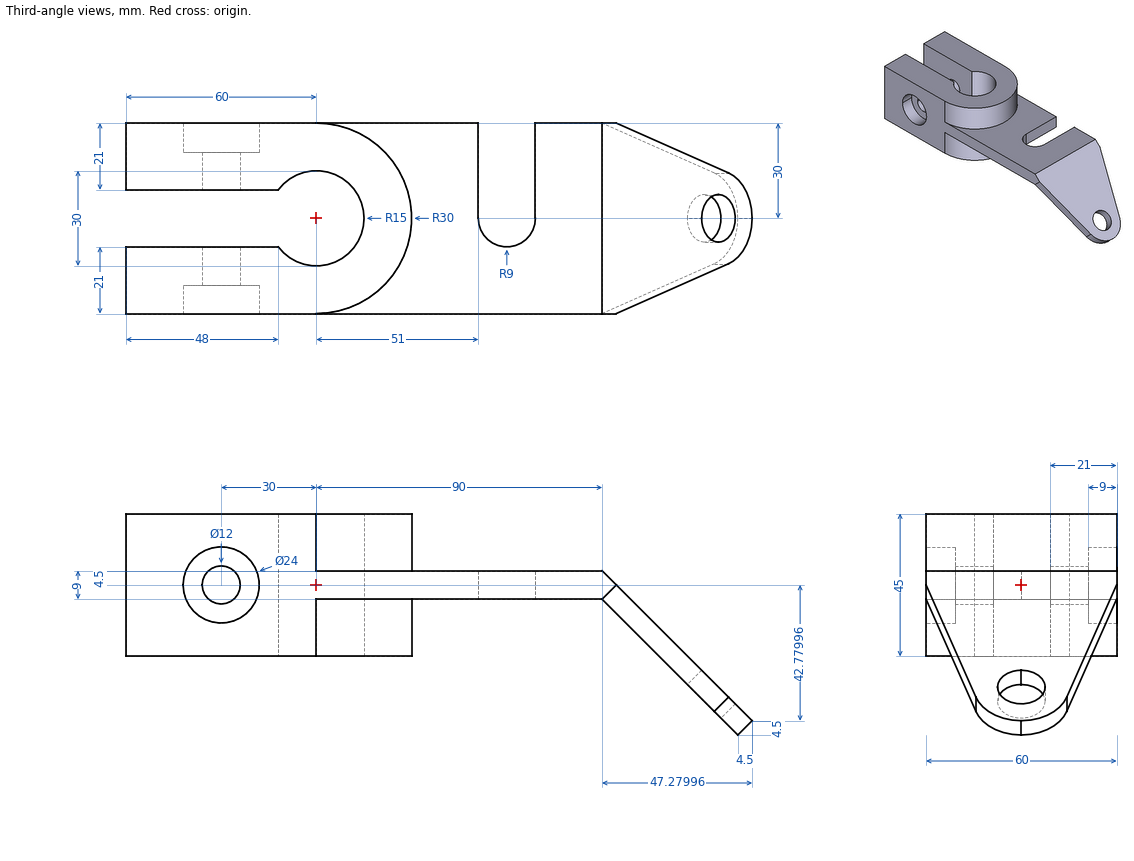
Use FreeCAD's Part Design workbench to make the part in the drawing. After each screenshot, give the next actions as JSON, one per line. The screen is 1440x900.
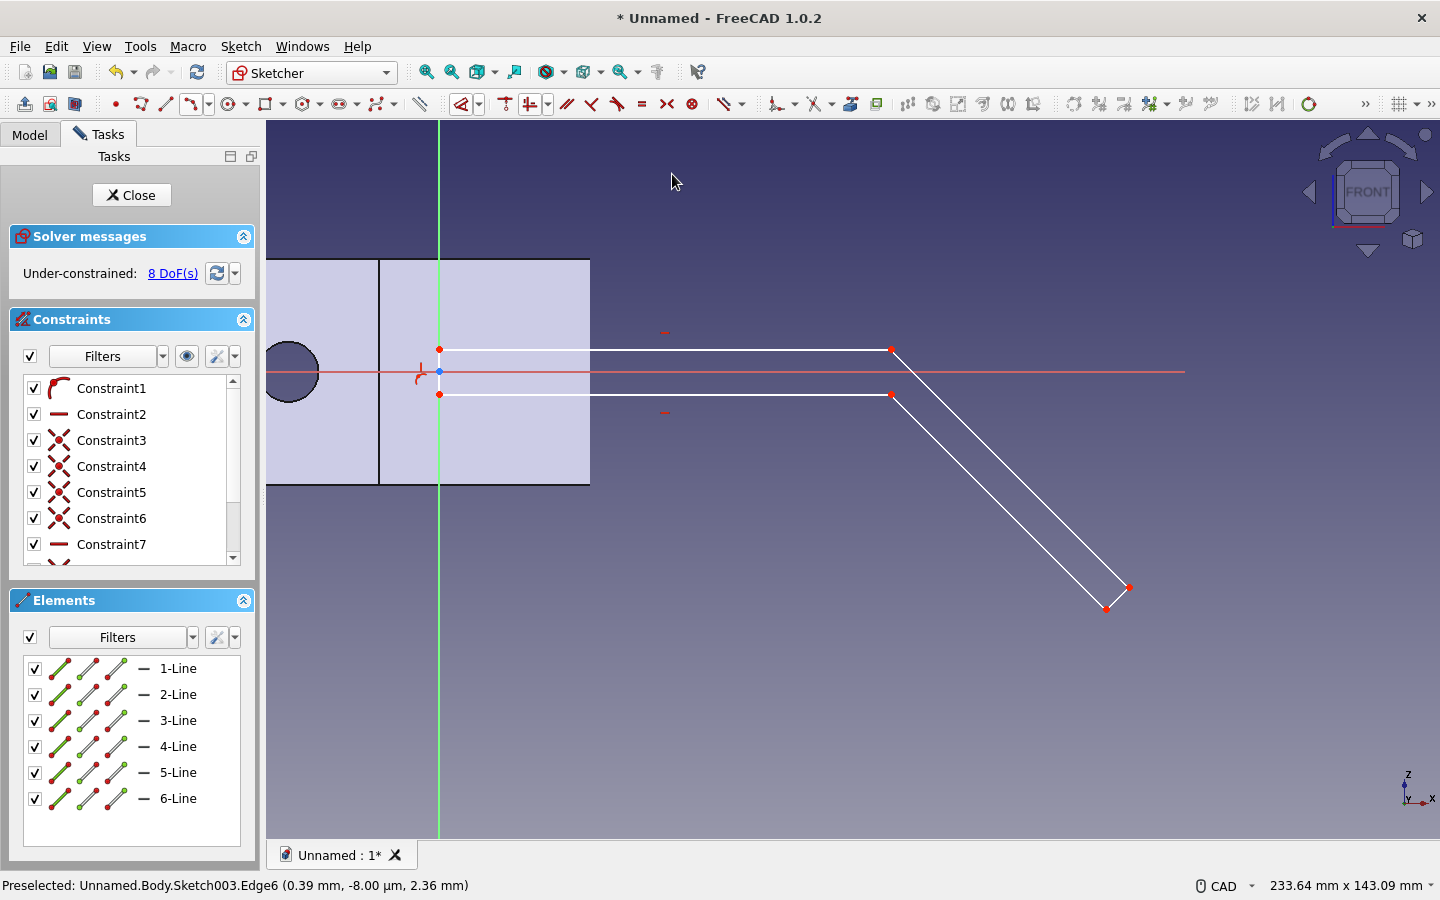
{"action": "scroll", "coordinate": [439, 382], "scroll_direction": "up", "scroll_amount": 2}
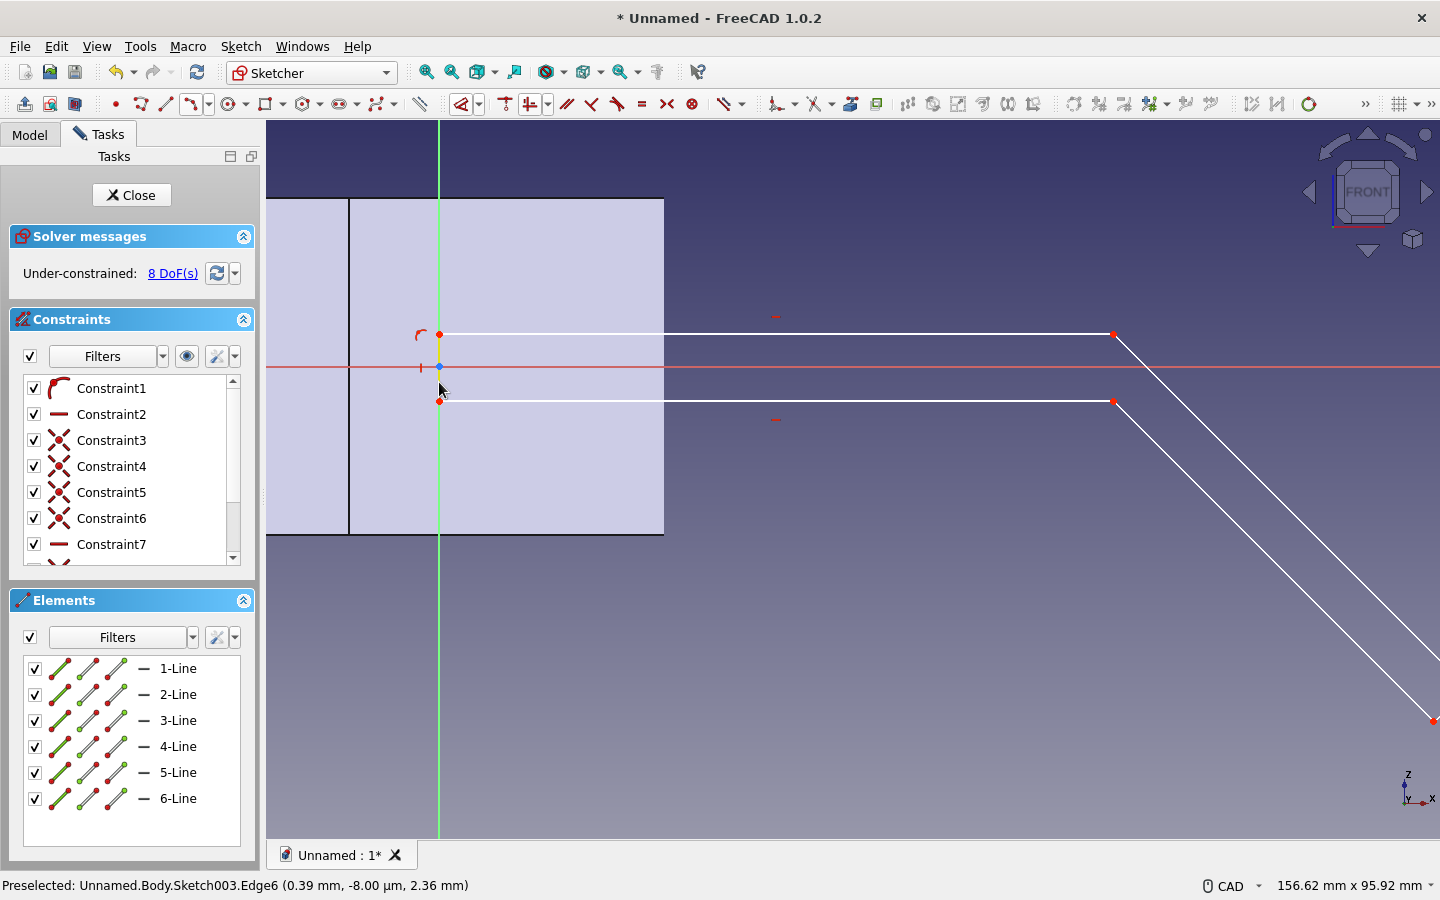
{"action": "left_click", "coordinate": [439, 381]}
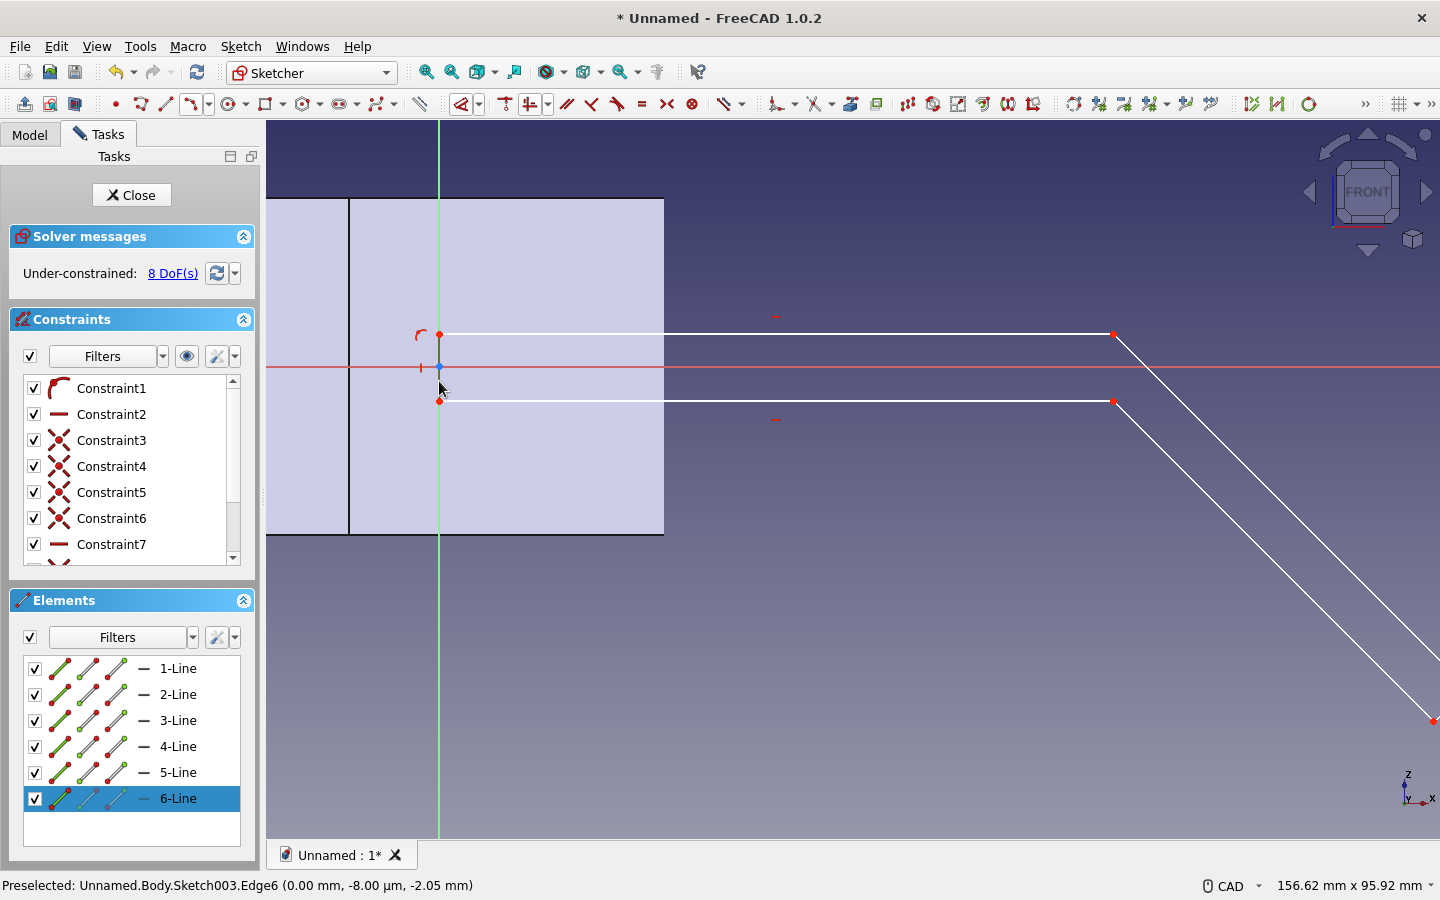
{"action": "left_click", "coordinate": [478, 104]}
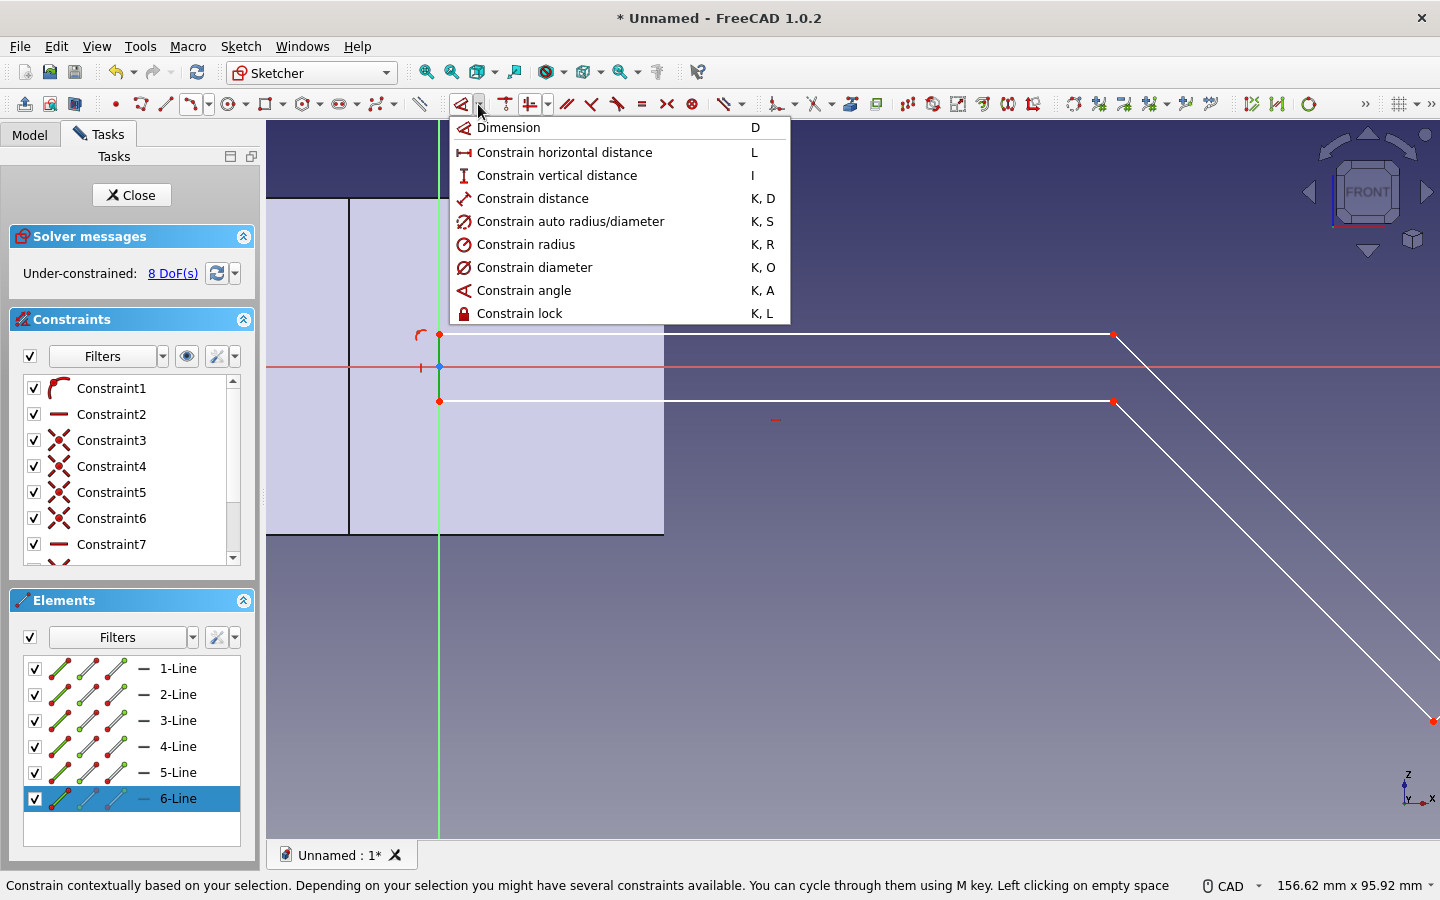
{"action": "left_click", "coordinate": [620, 176]}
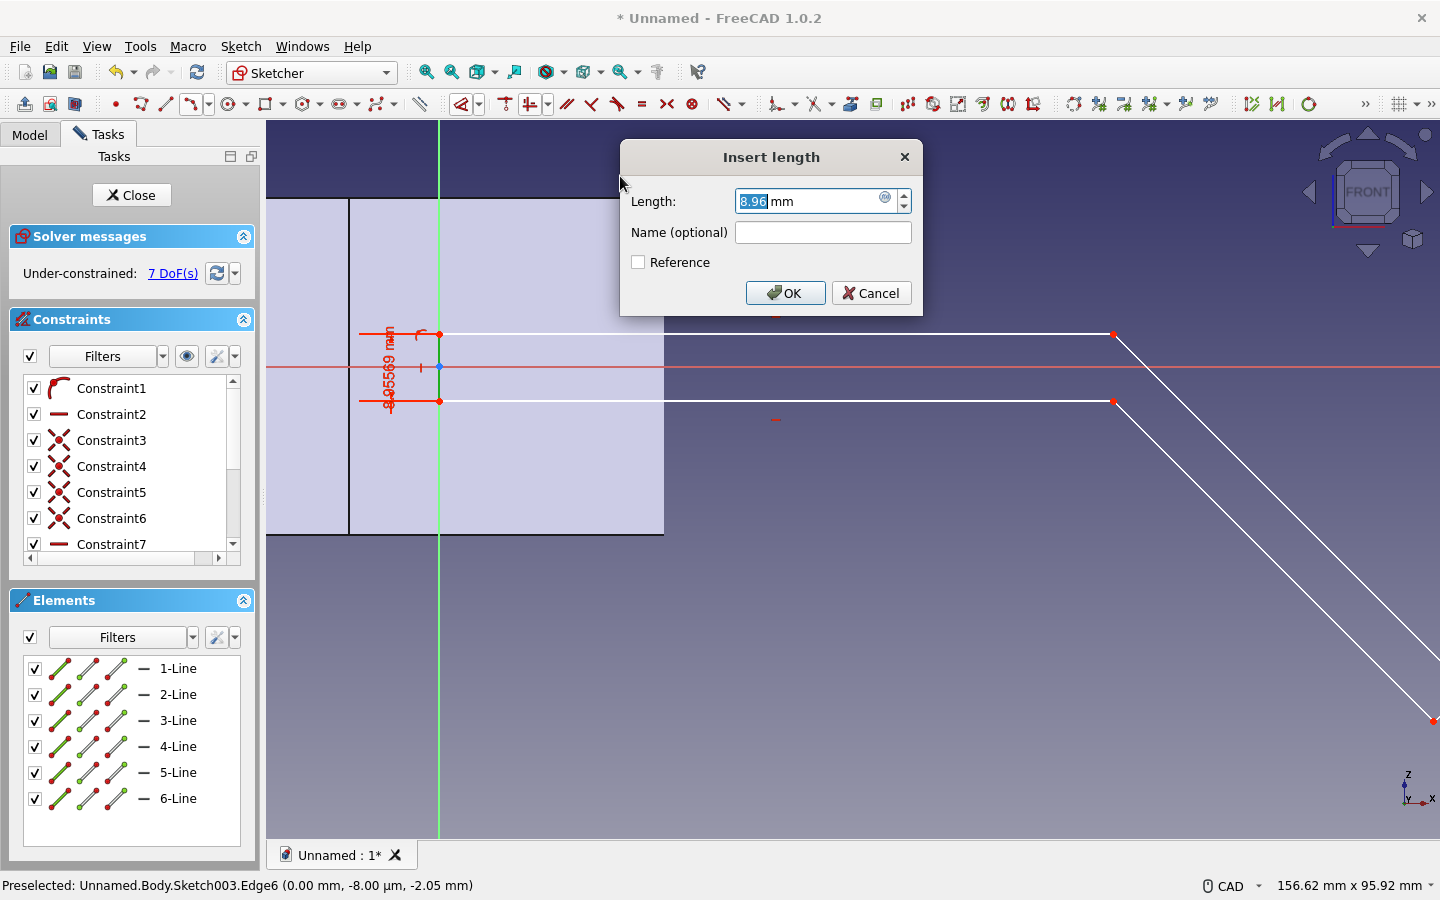
{"action": "type", "text": "9"}
{"action": "key", "text": "Return"}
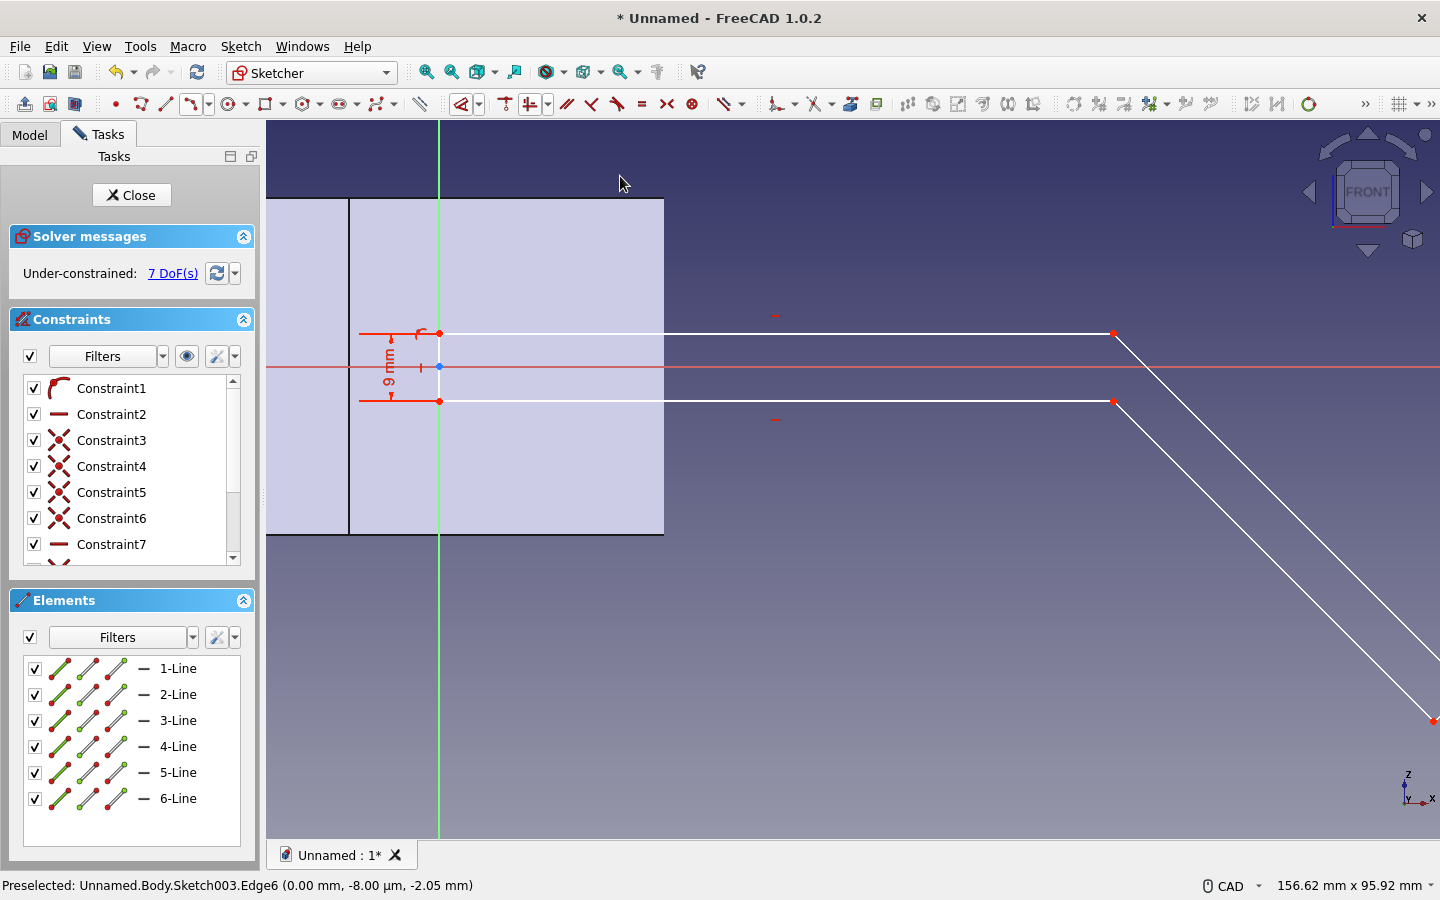
{"action": "left_click", "coordinate": [641, 334]}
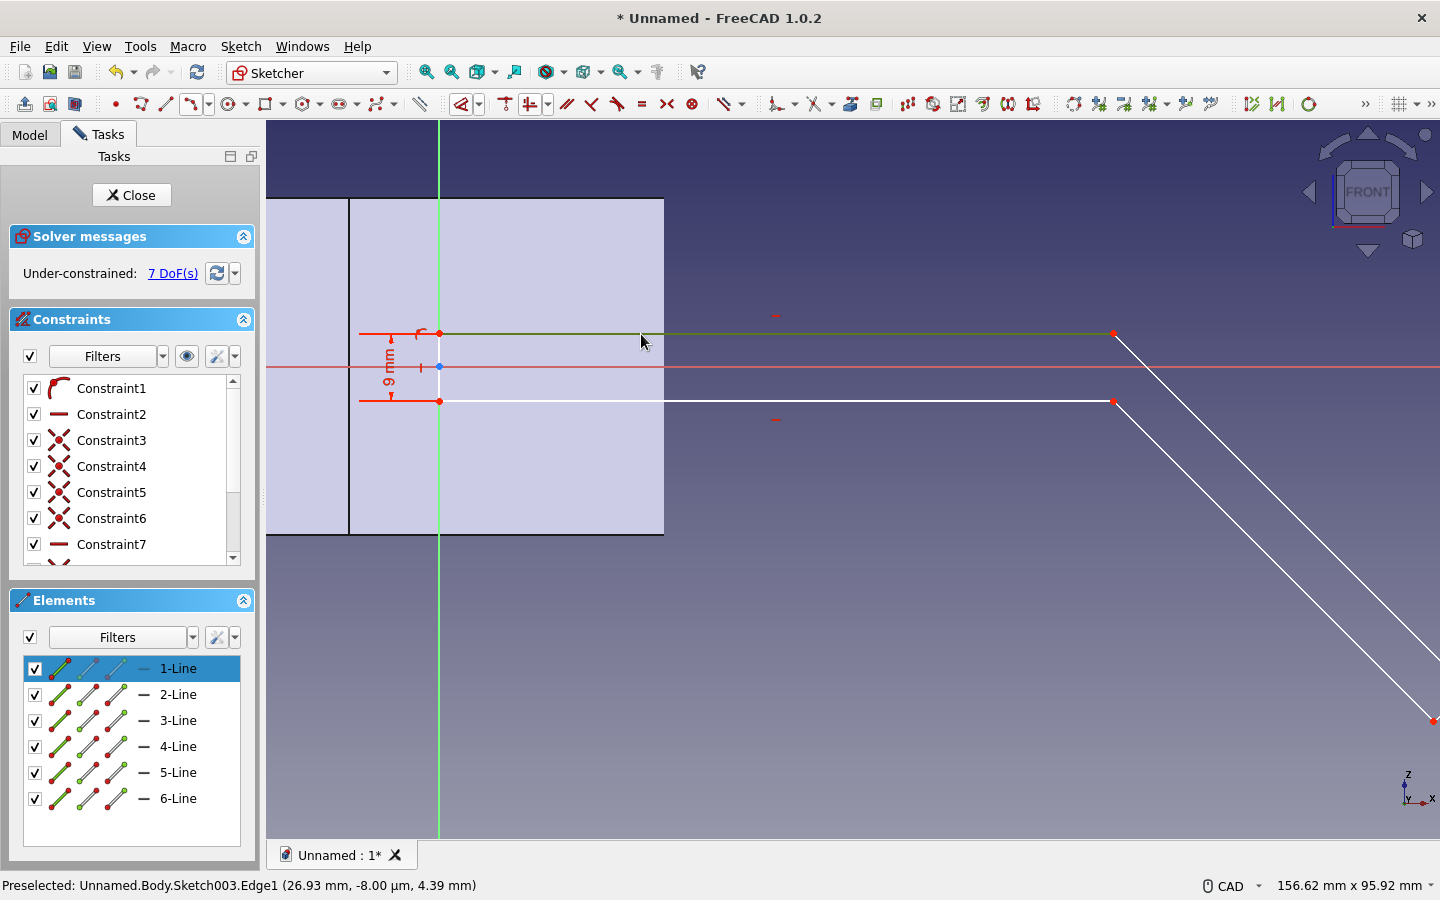
{"action": "left_click", "coordinate": [478, 104]}